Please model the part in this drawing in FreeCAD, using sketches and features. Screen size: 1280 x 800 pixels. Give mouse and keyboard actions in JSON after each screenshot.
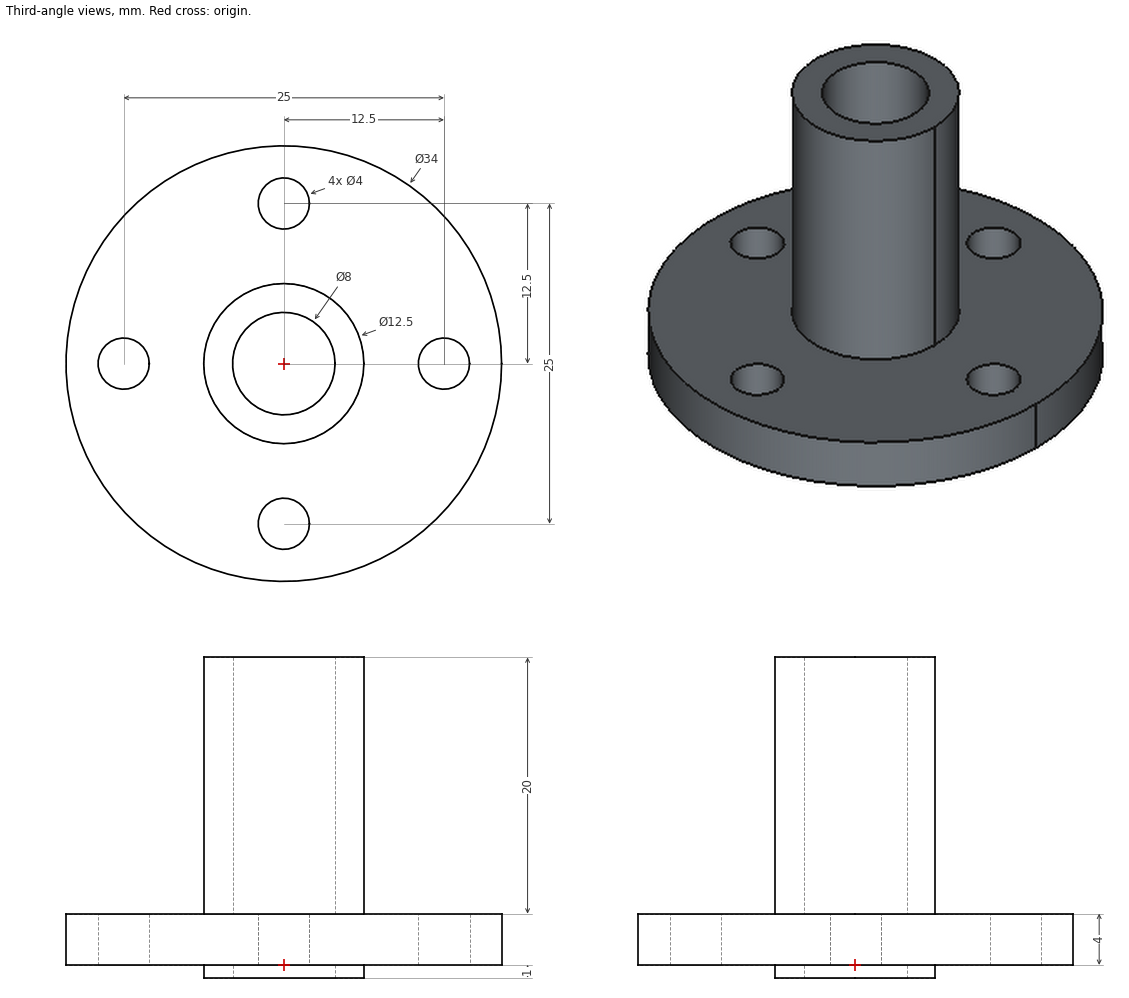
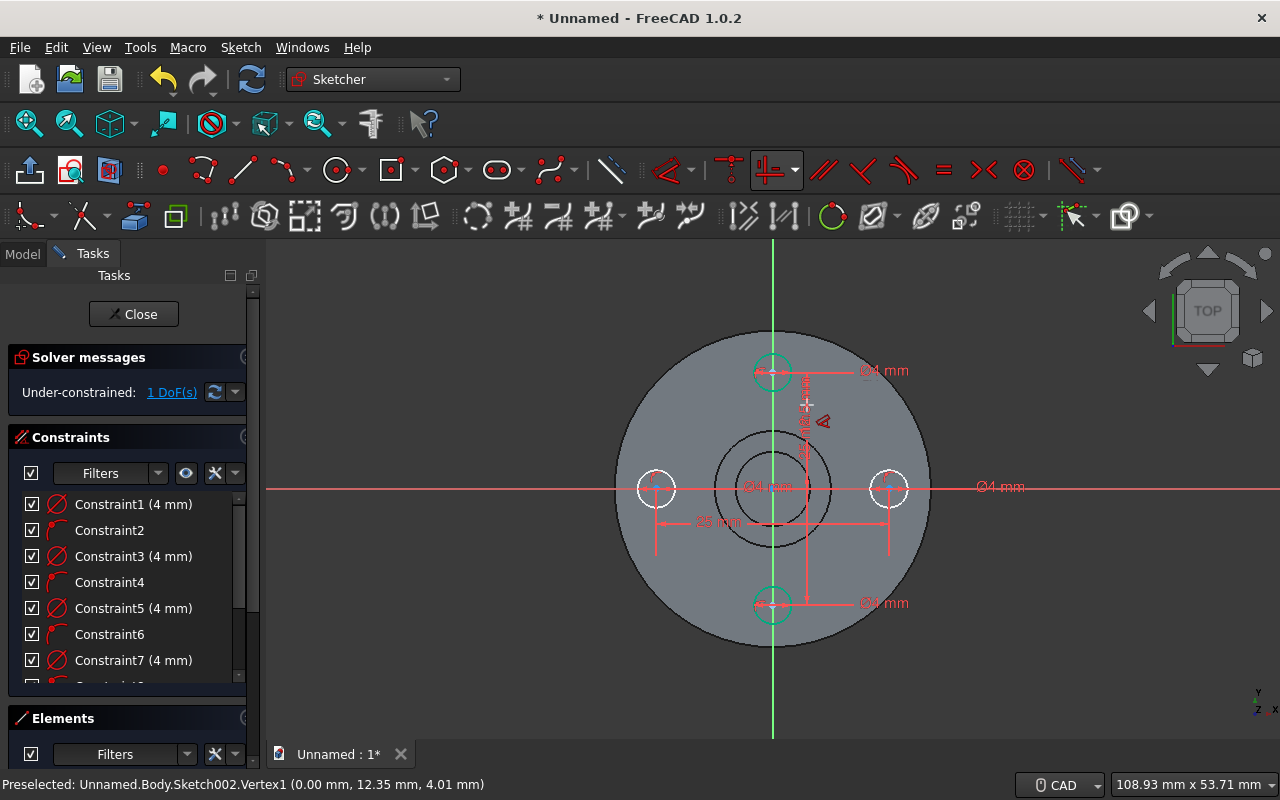
{"action": "left_click", "coordinate": [889, 489]}
{"action": "left_click", "coordinate": [831, 523]}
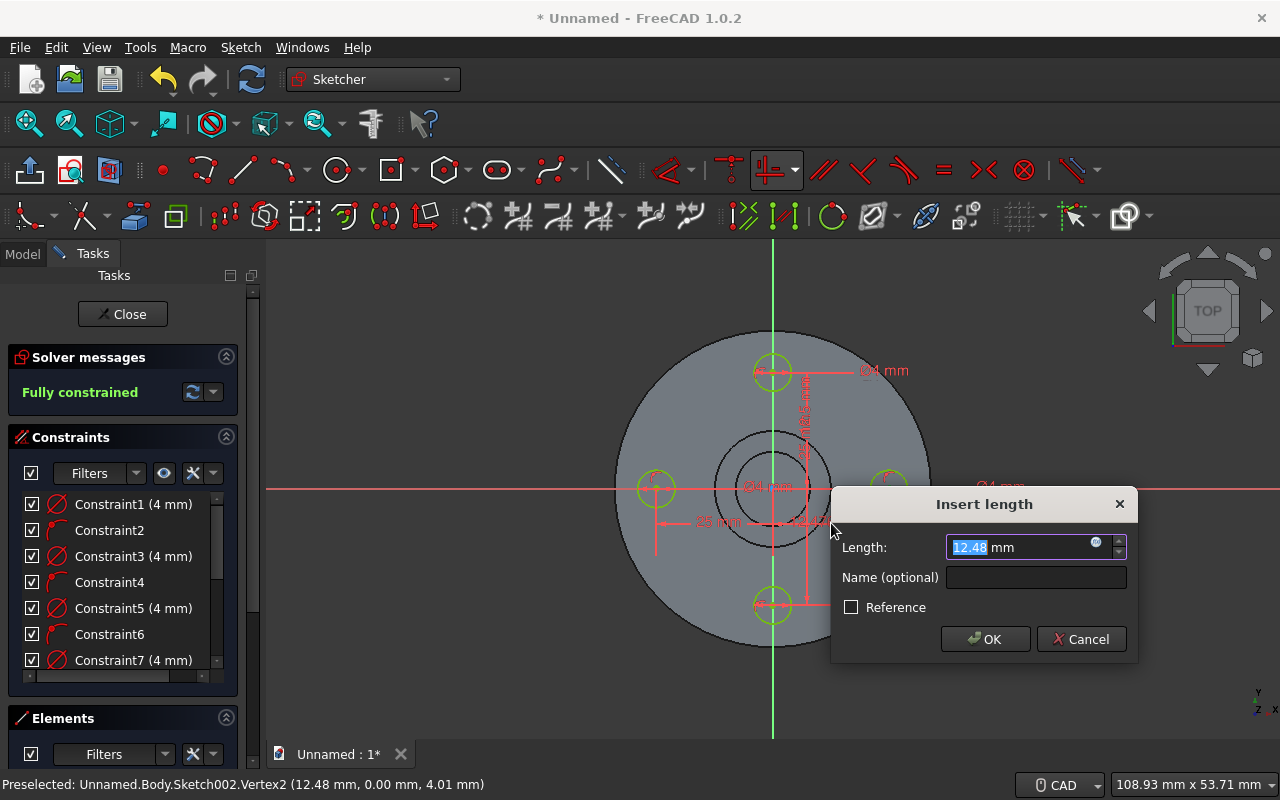
{"action": "type", "text": "12.5"}
{"action": "key", "text": "Return"}
{"action": "key", "text": "Escape"}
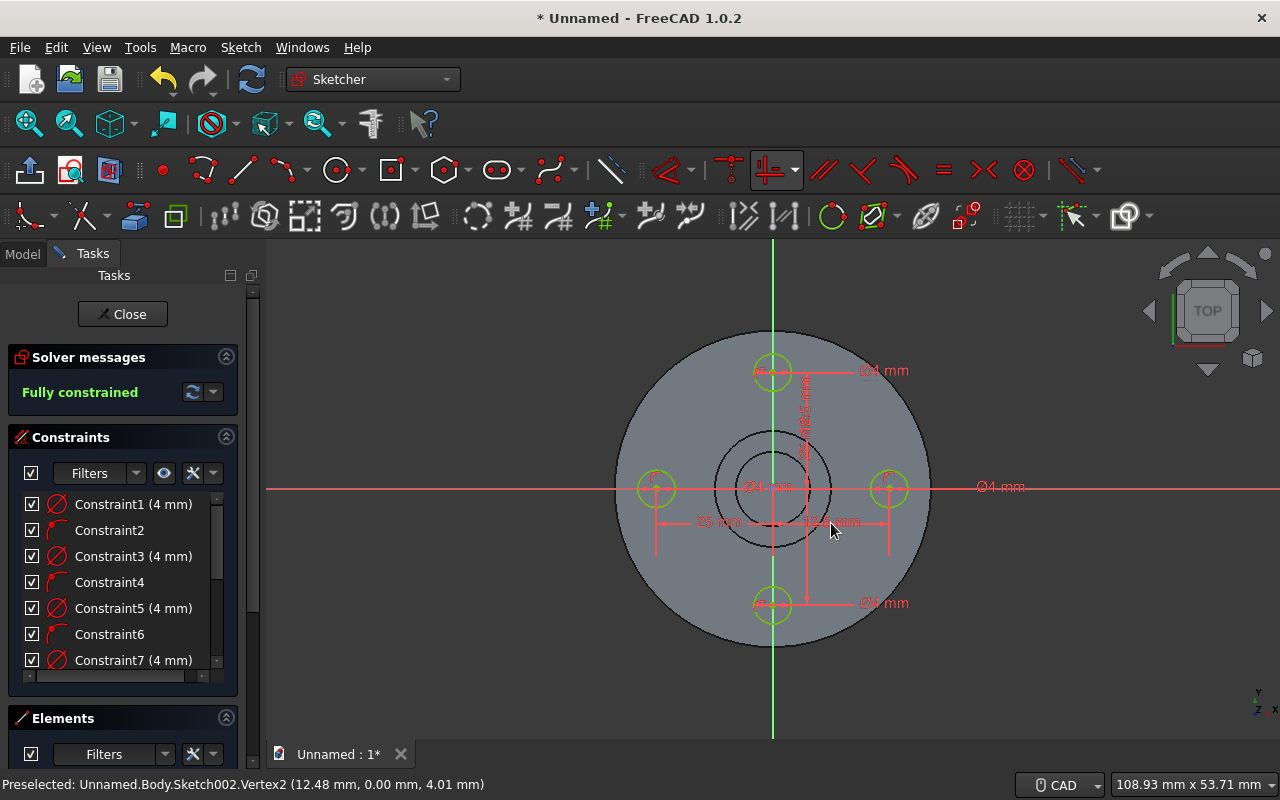
{"action": "left_click", "coordinate": [123, 314]}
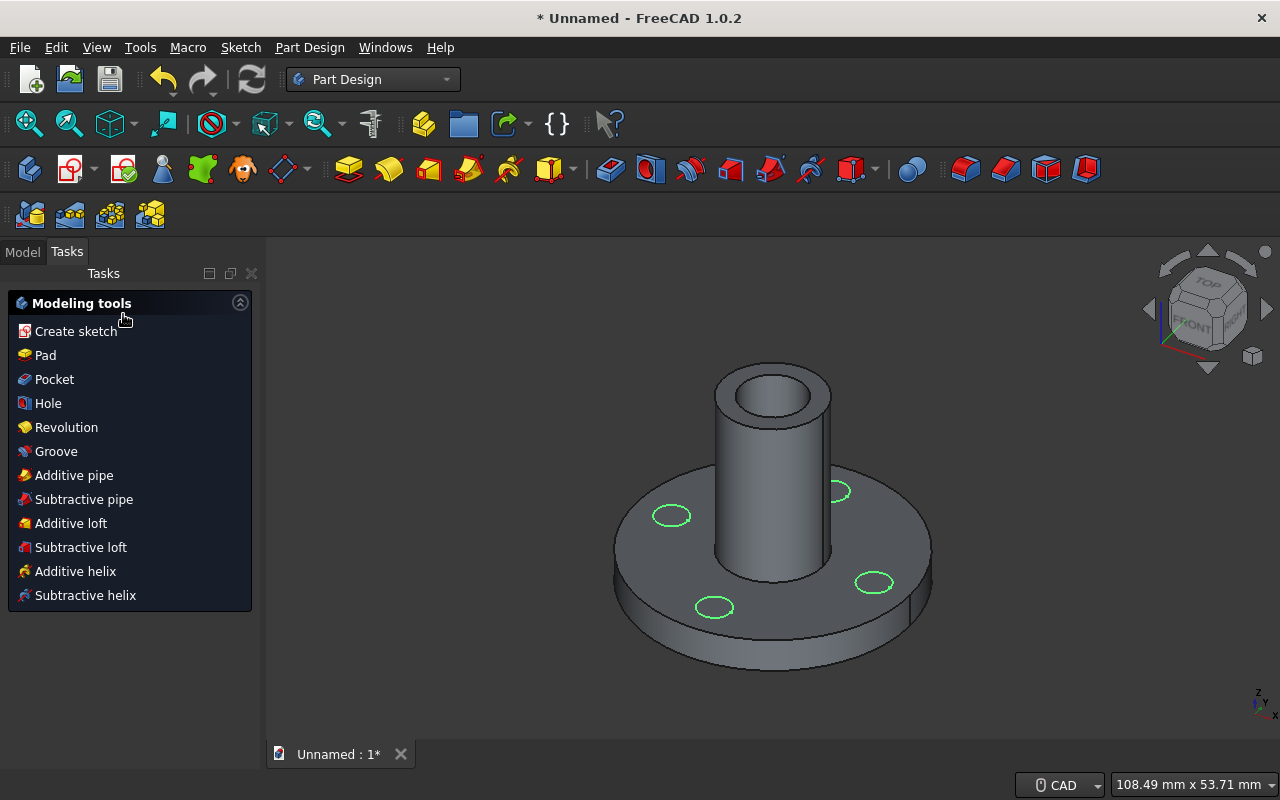
{"action": "left_click", "coordinate": [612, 170]}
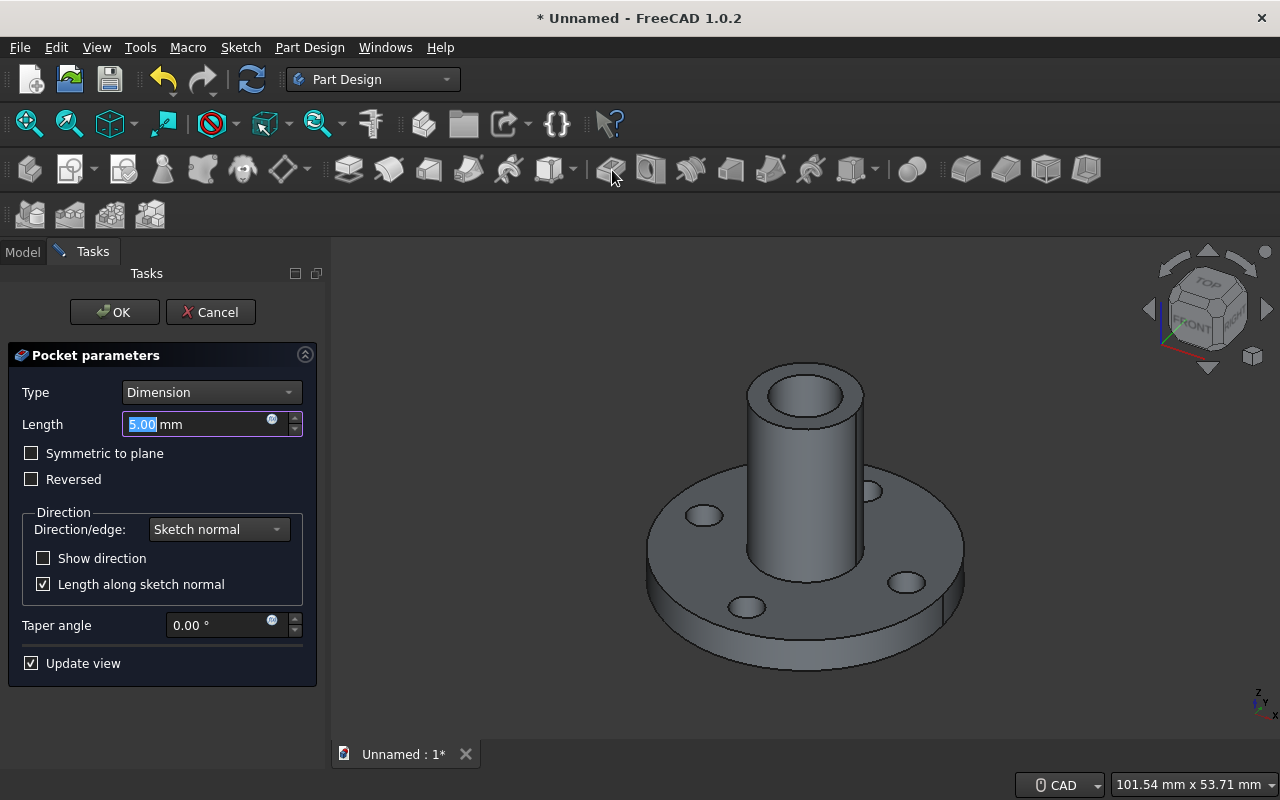
{"action": "type", "text": "4"}
{"action": "key", "text": "Tab"}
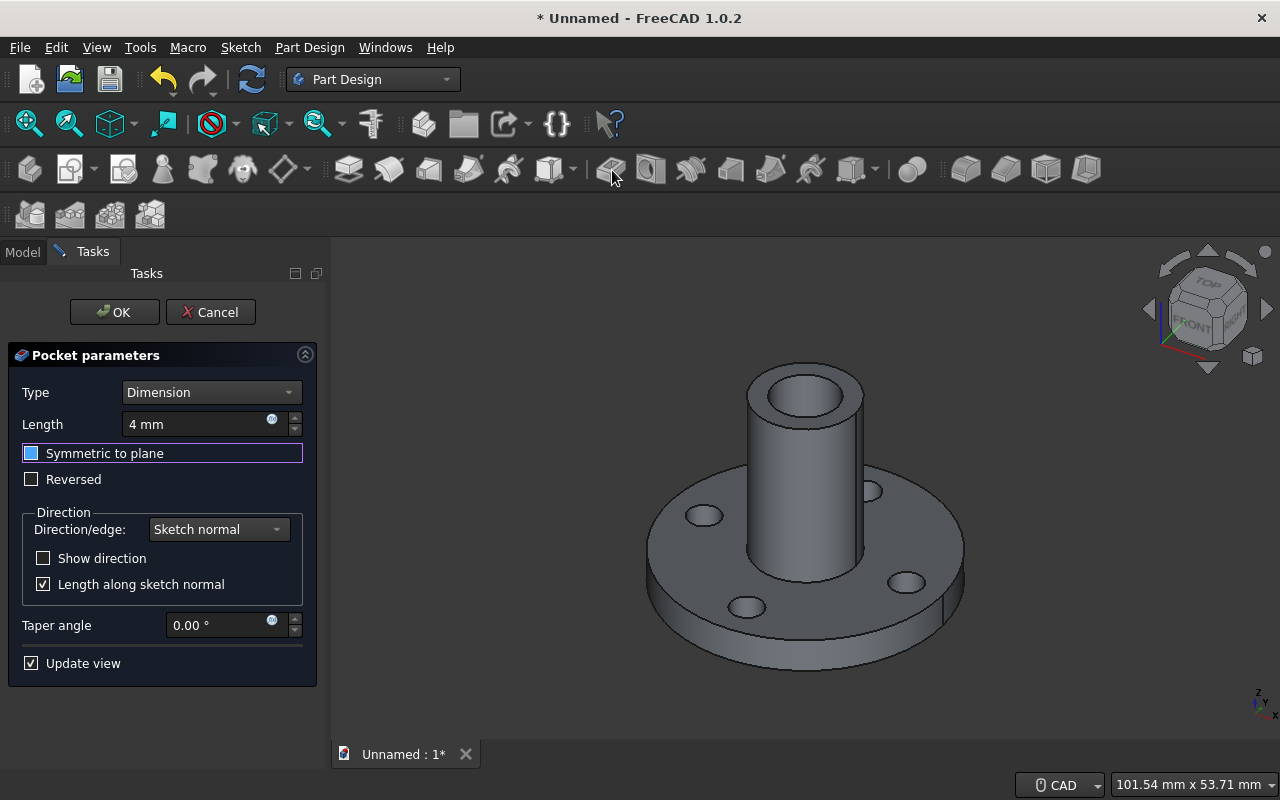
{"action": "left_click", "coordinate": [115, 312]}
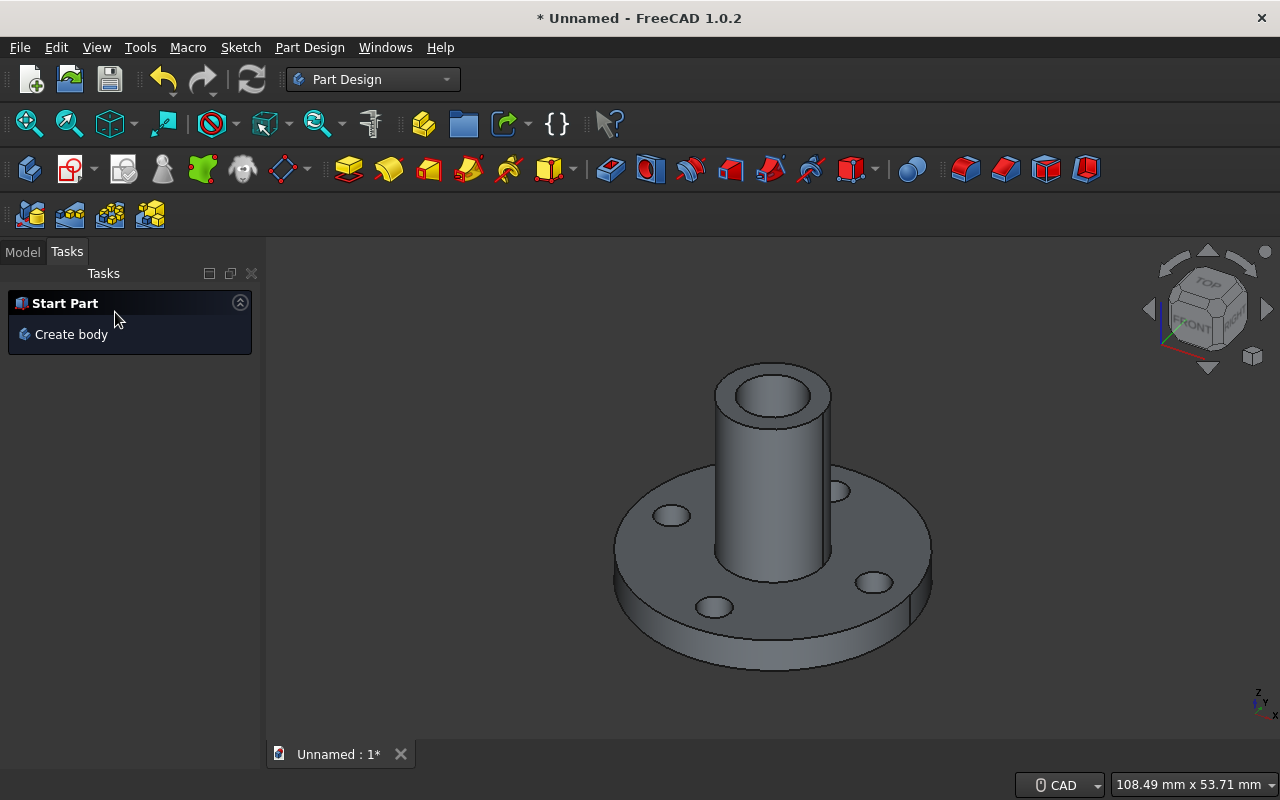
{"action": "left_click", "coordinate": [23, 251]}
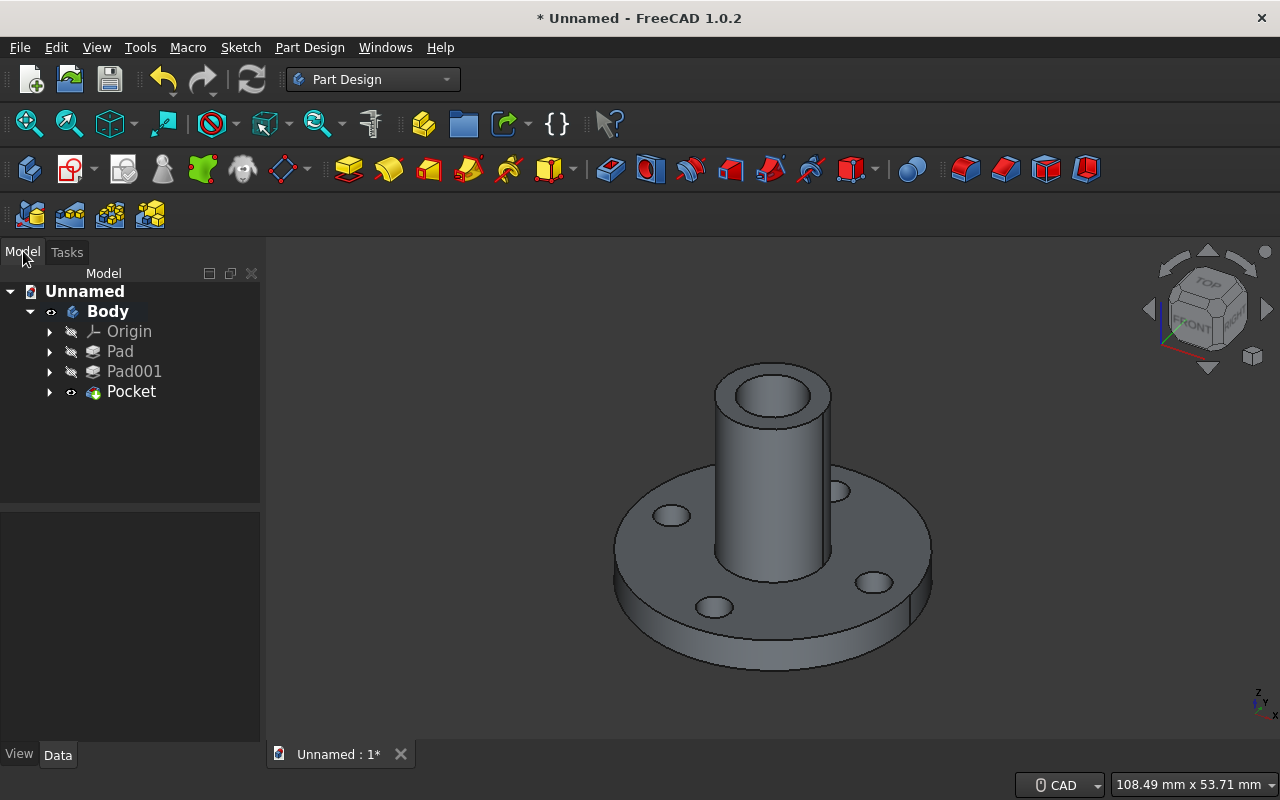
{"action": "left_click", "coordinate": [50, 332]}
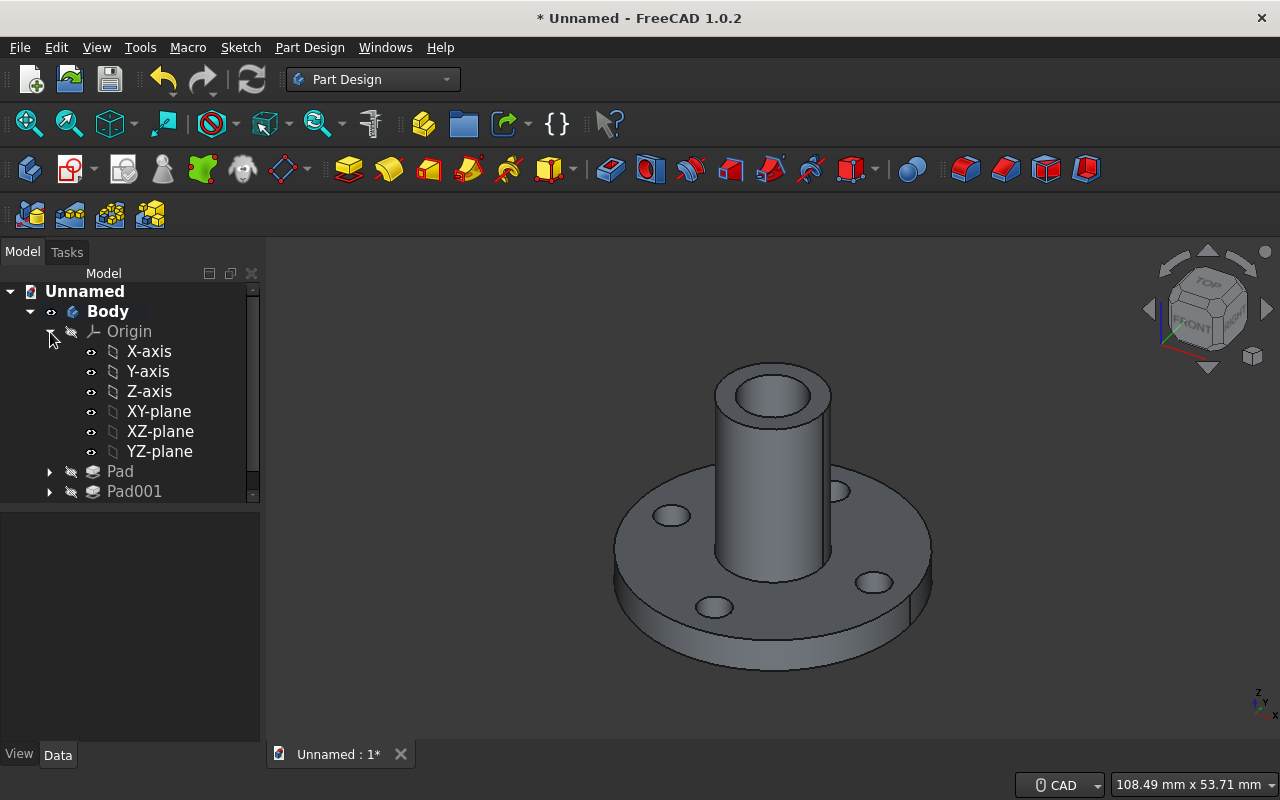
{"action": "left_click", "coordinate": [136, 412]}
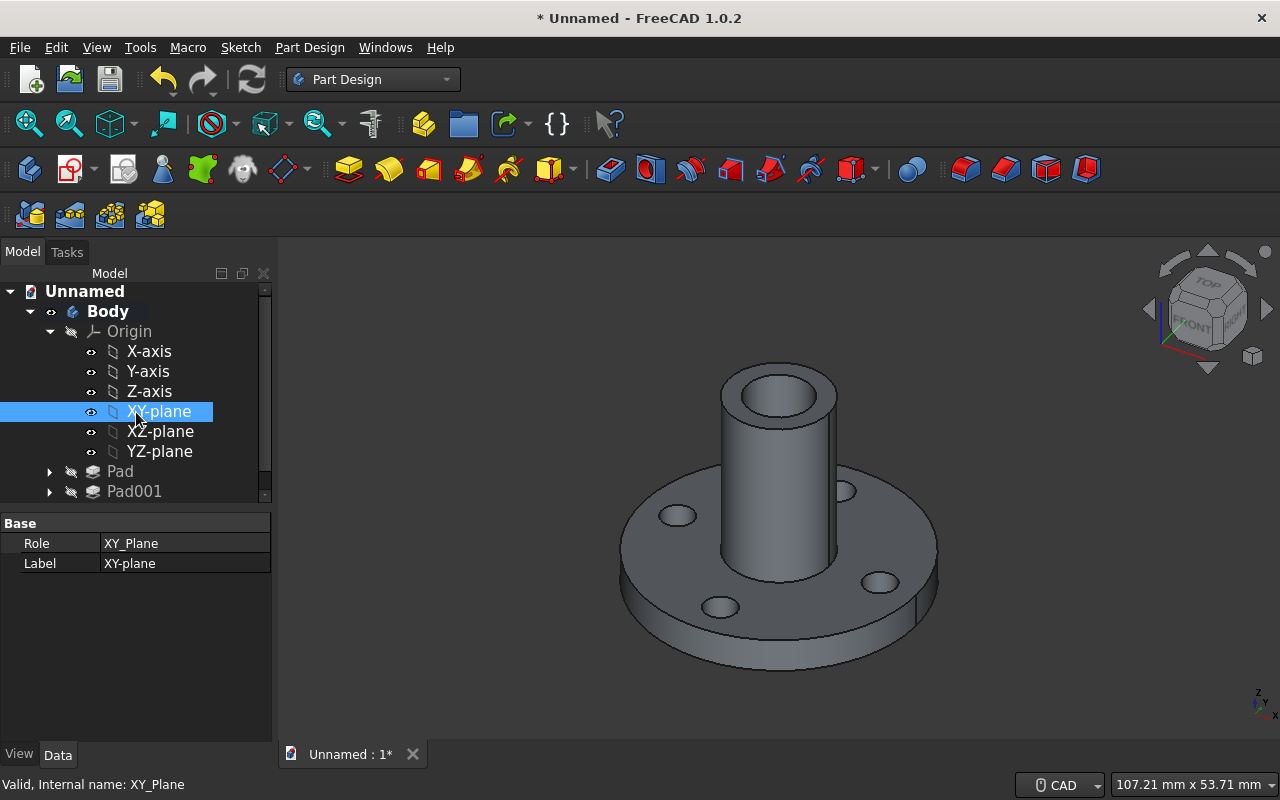
{"action": "left_click", "coordinate": [284, 170]}